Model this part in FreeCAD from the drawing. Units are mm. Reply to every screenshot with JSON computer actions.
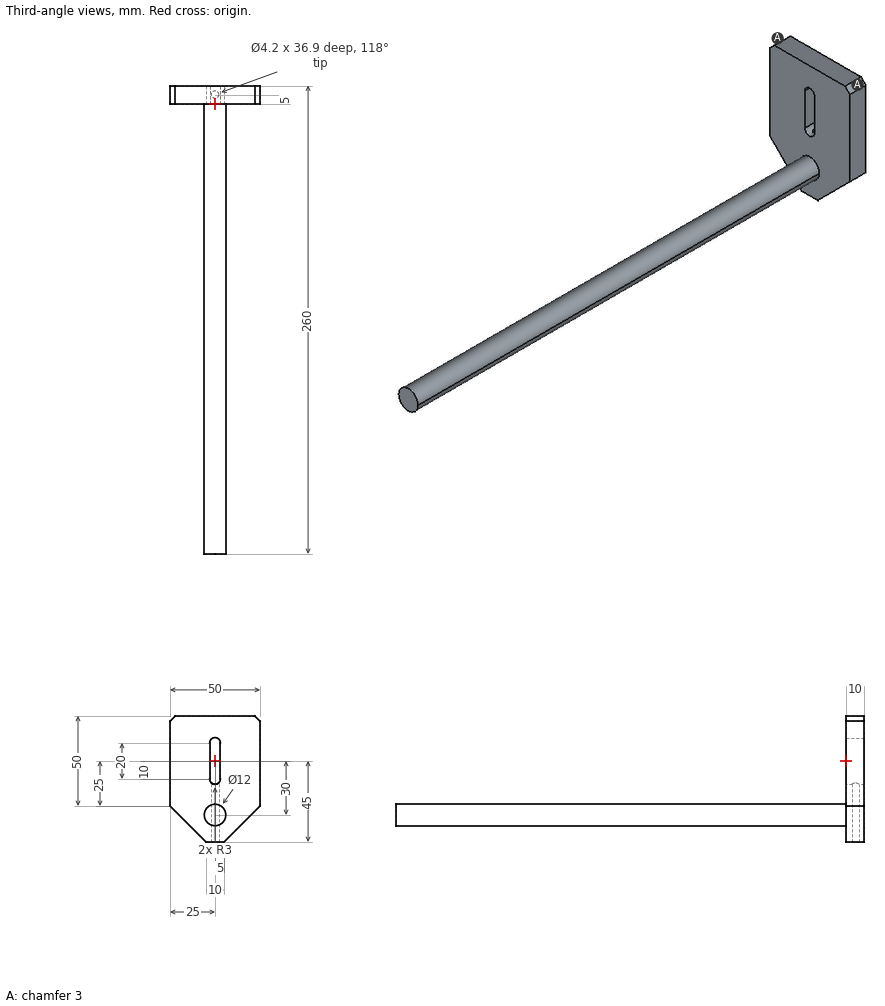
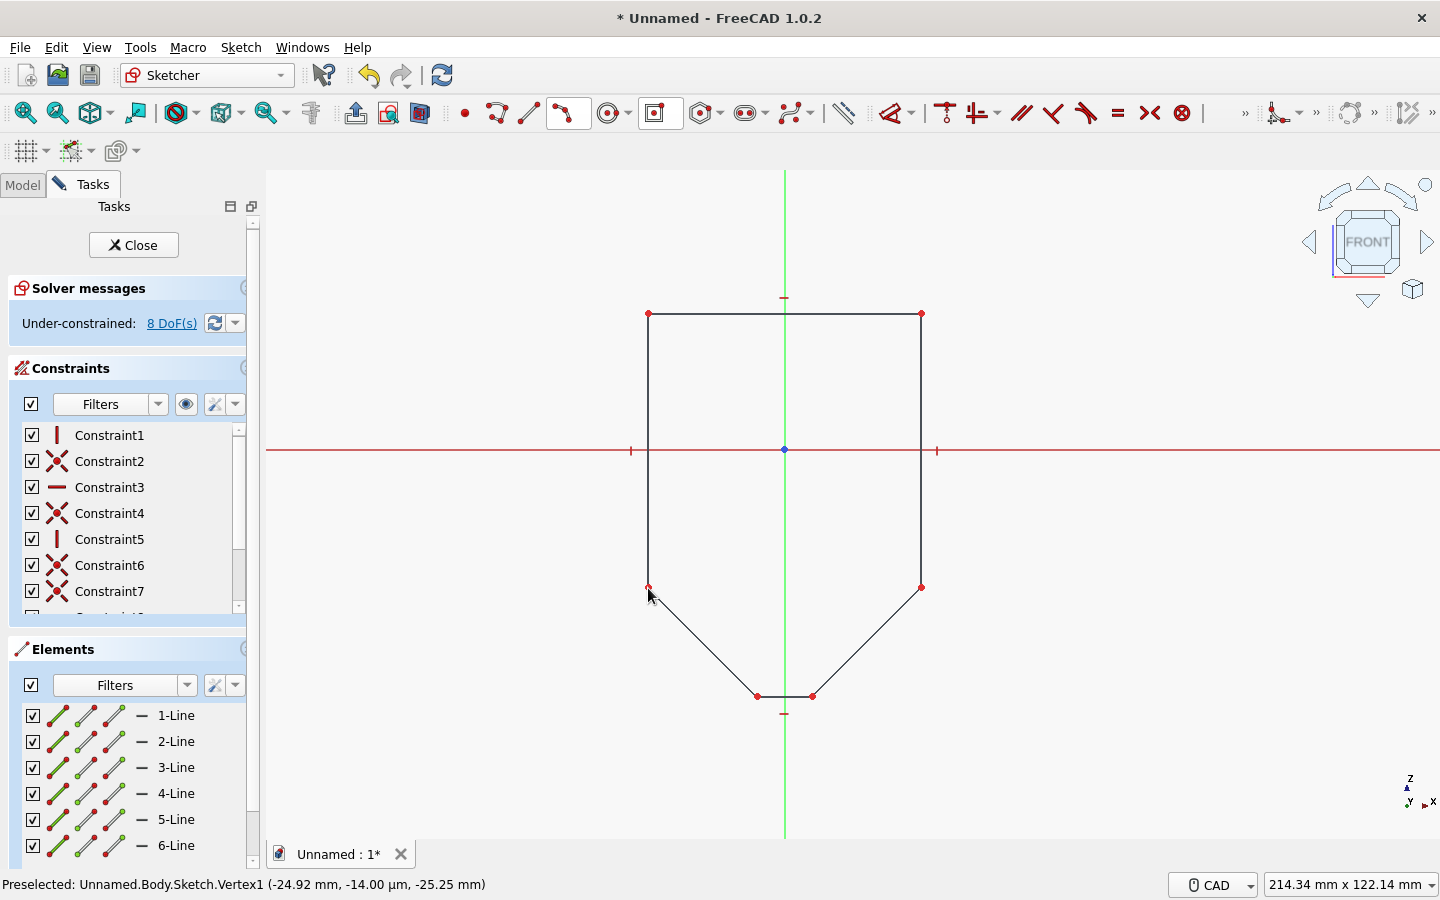
{"action": "left_click", "coordinate": [648, 506]}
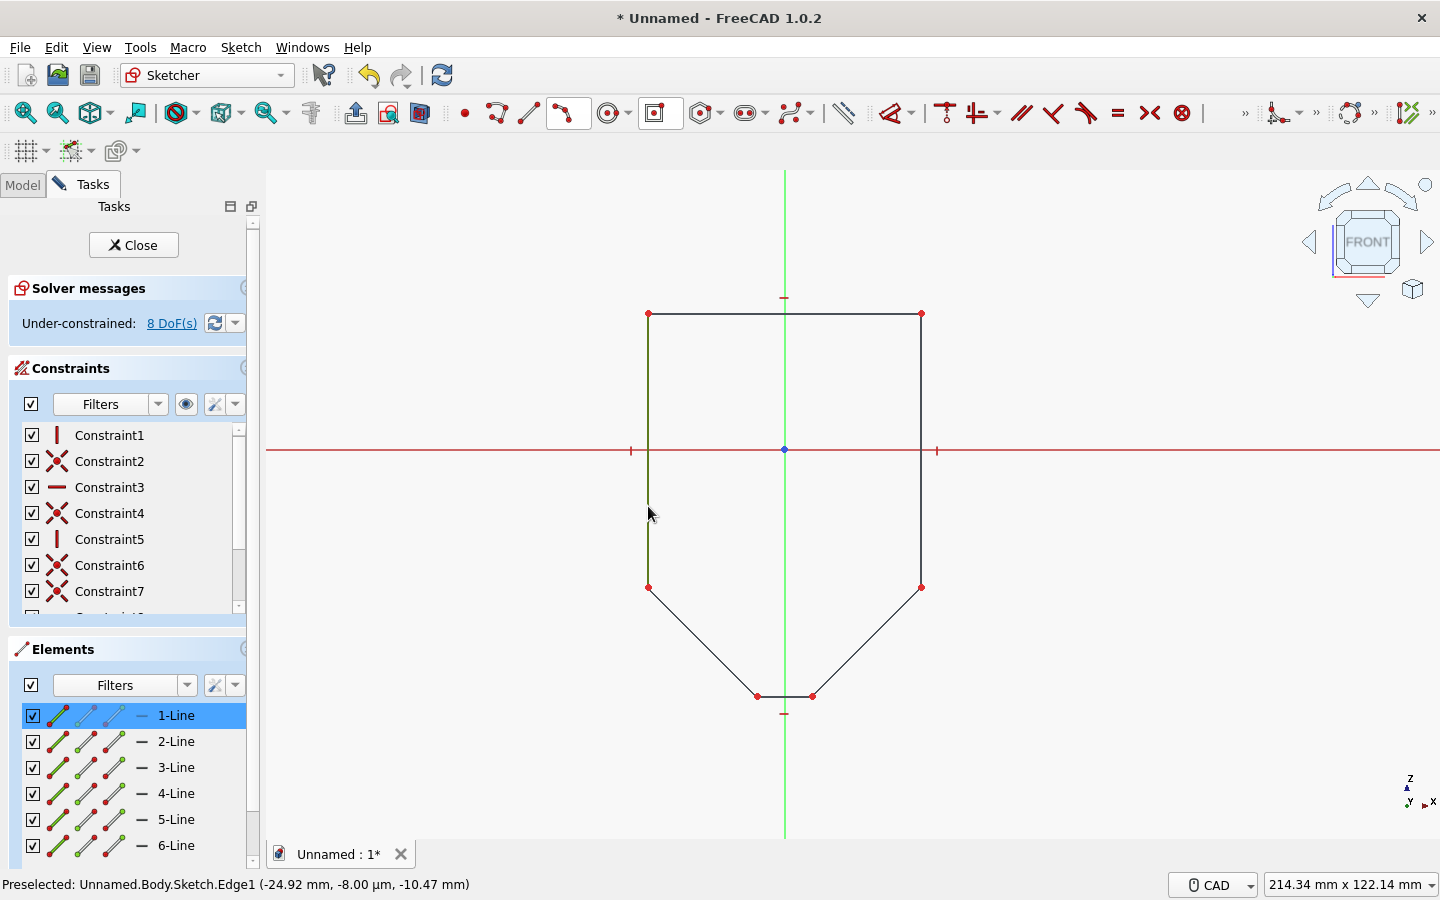
{"action": "key", "text": "i"}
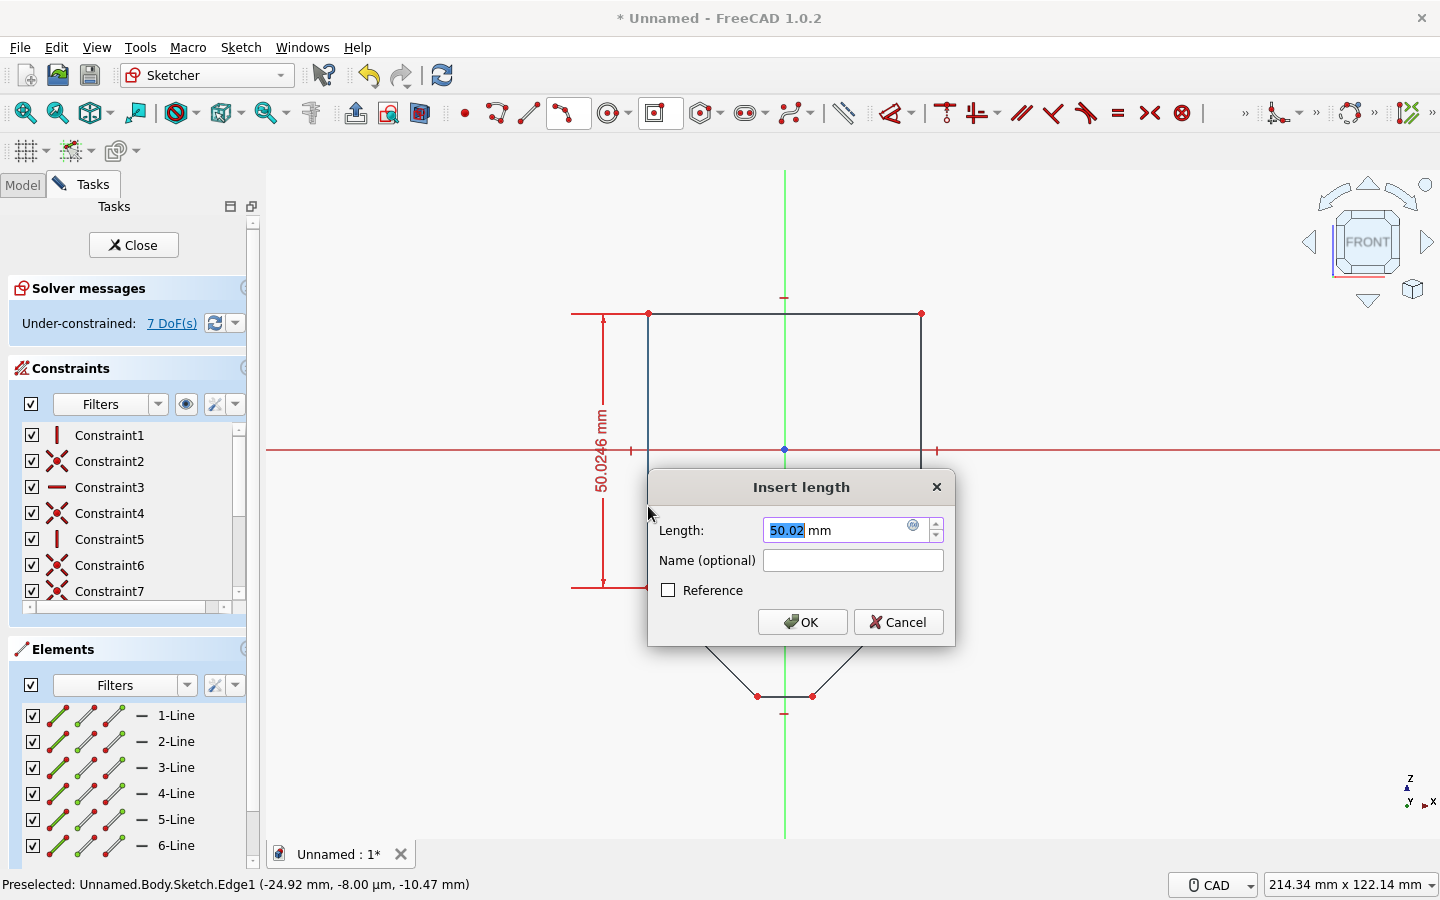
{"action": "type", "text": "50"}
{"action": "key", "text": "Return"}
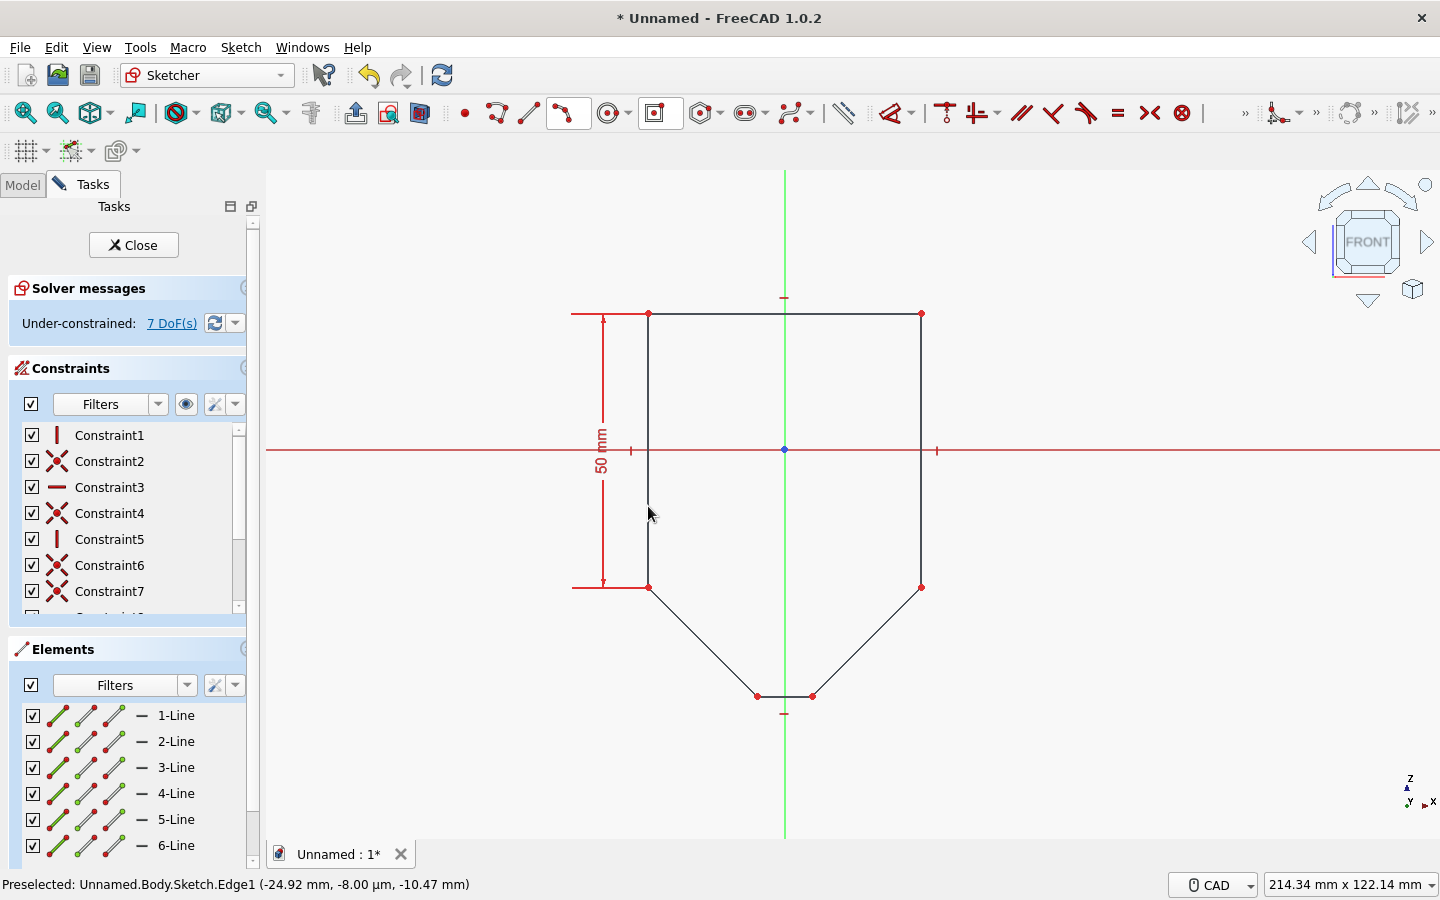
{"action": "left_click", "coordinate": [730, 314]}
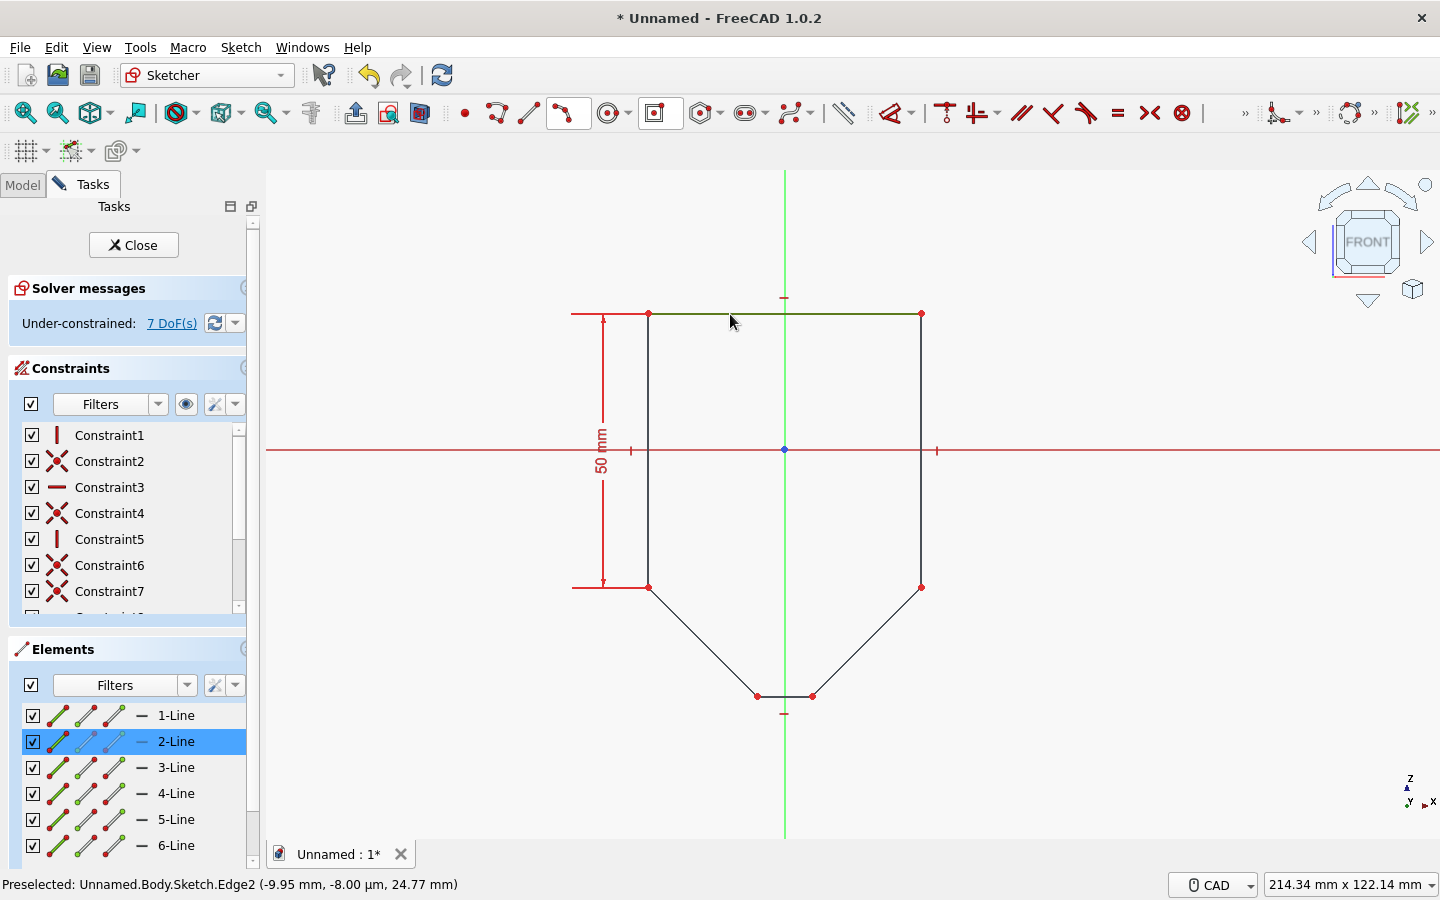
{"action": "key", "text": "l"}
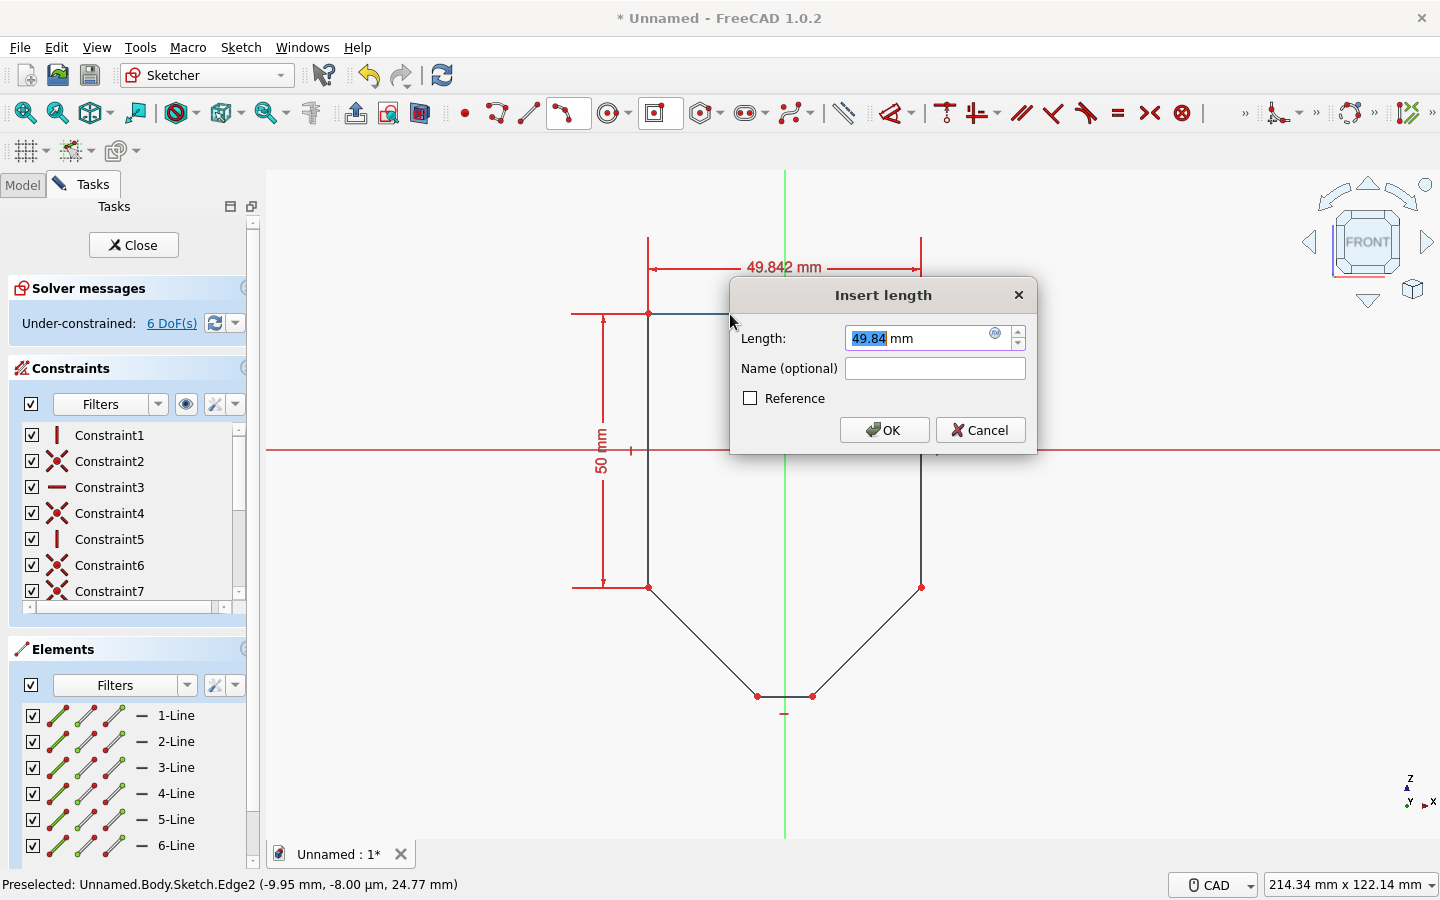
{"action": "type", "text": "50"}
{"action": "key", "text": "Return"}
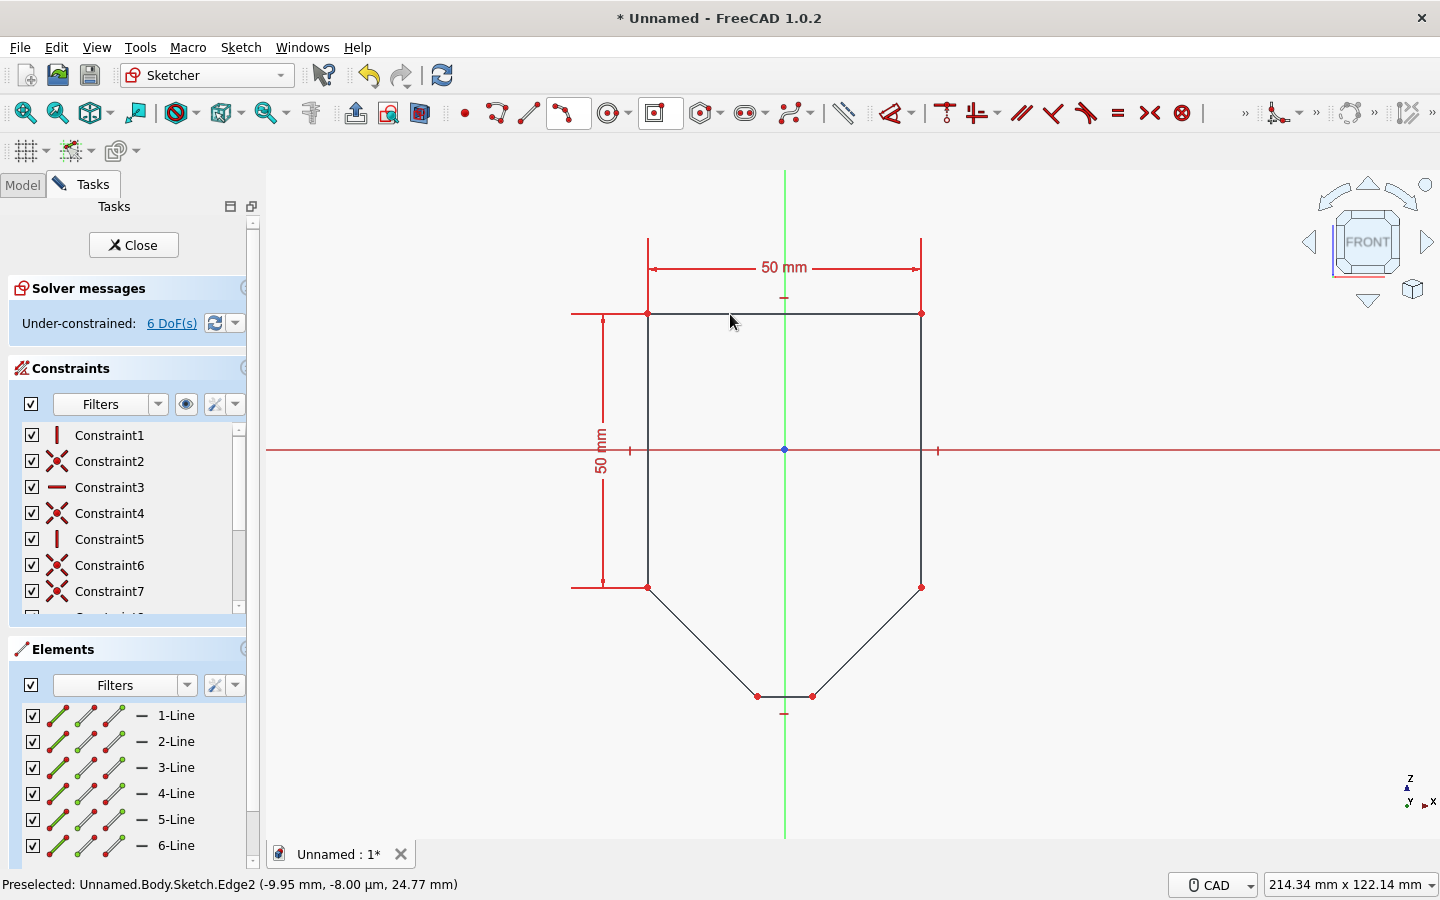
{"action": "left_click", "coordinate": [921, 396]}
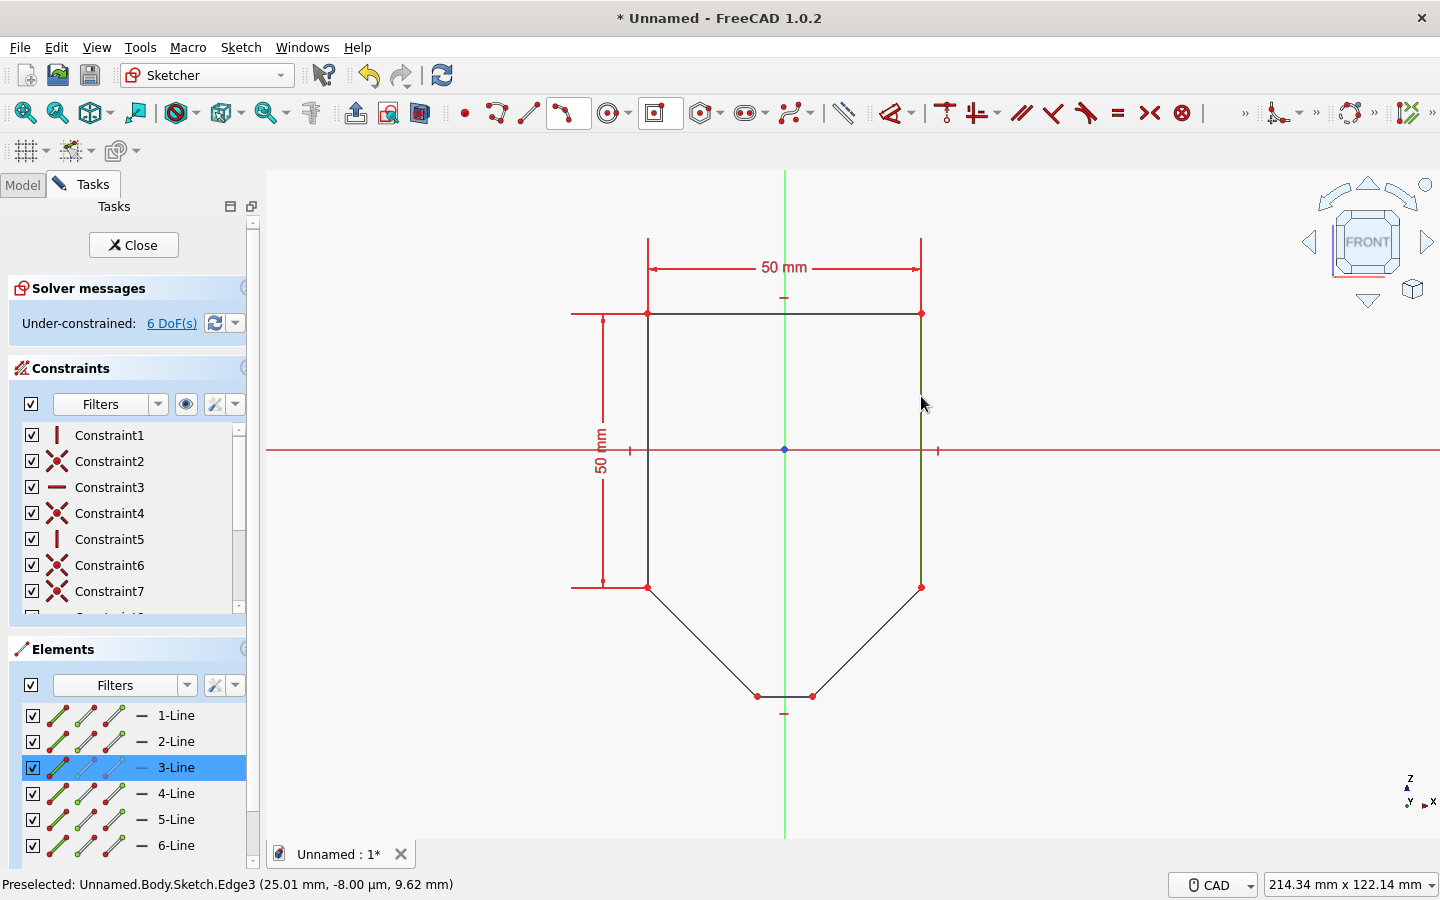
{"action": "left_click", "coordinate": [914, 114]}